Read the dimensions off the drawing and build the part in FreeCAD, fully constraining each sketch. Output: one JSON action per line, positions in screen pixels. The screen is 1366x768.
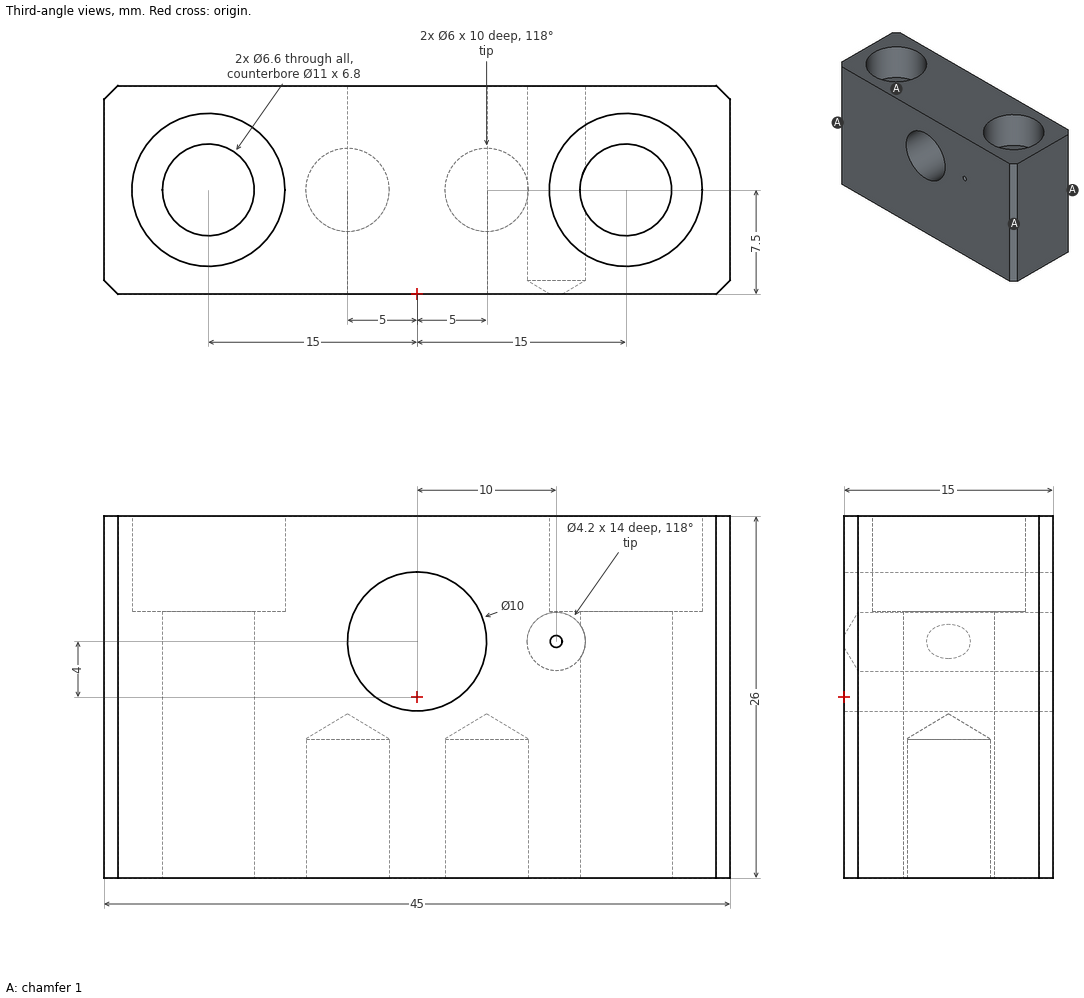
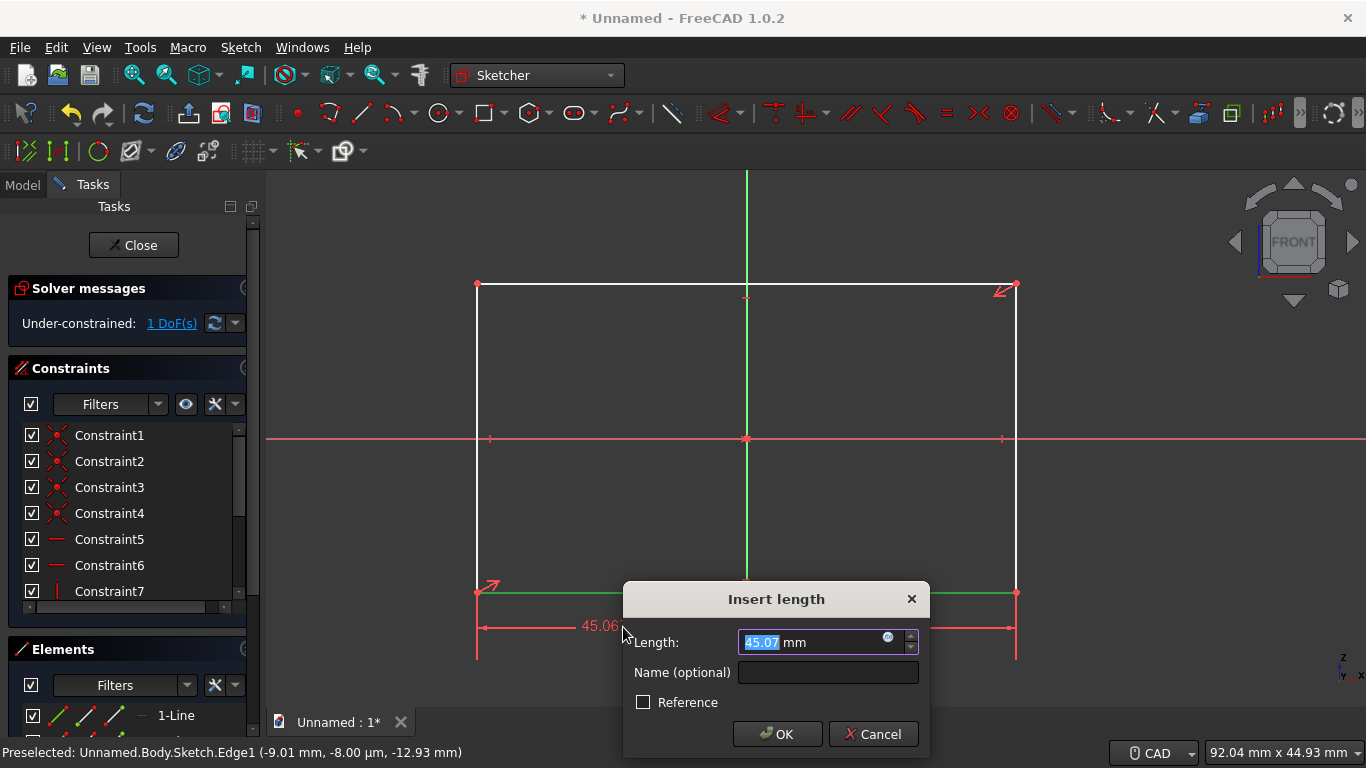
{"action": "type", "text": "45"}
{"action": "key", "text": "Return"}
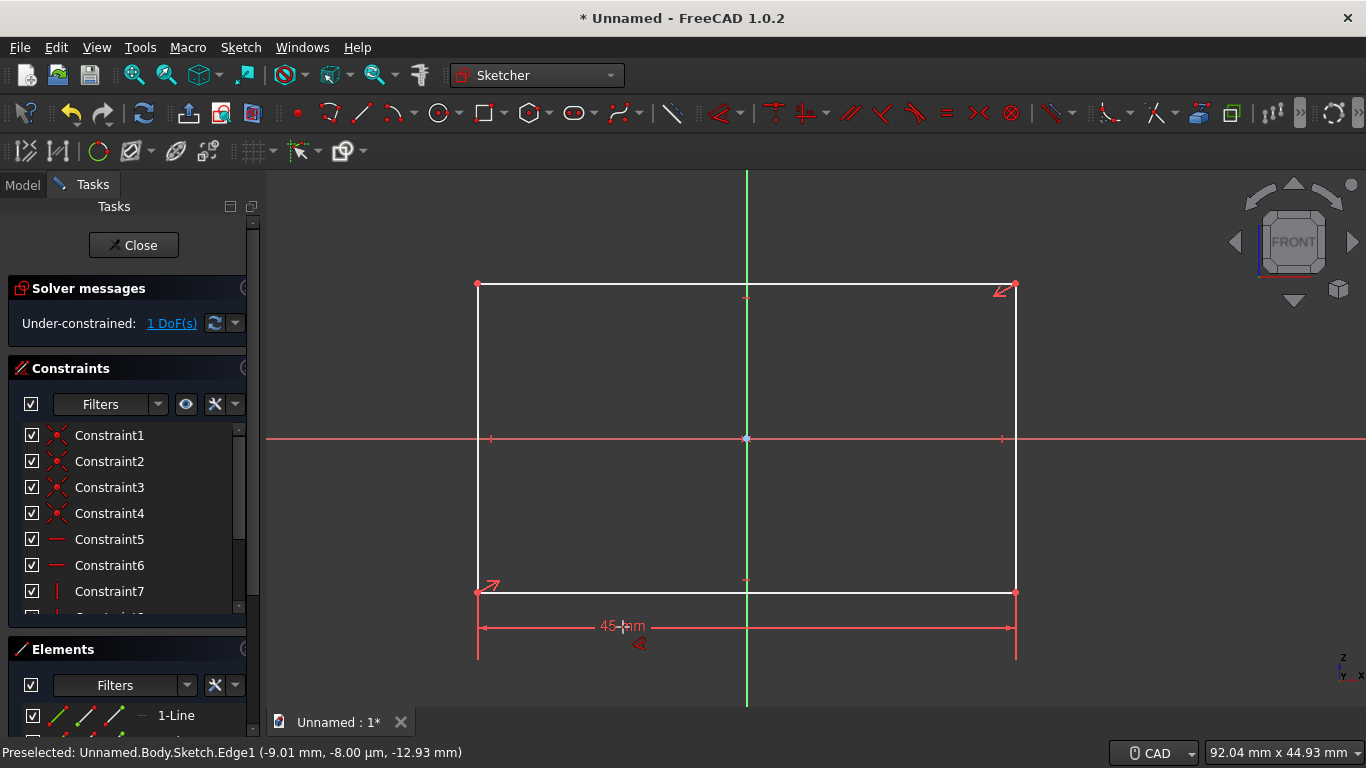
{"action": "left_click", "coordinate": [1016, 500]}
{"action": "left_click", "coordinate": [1050, 367]}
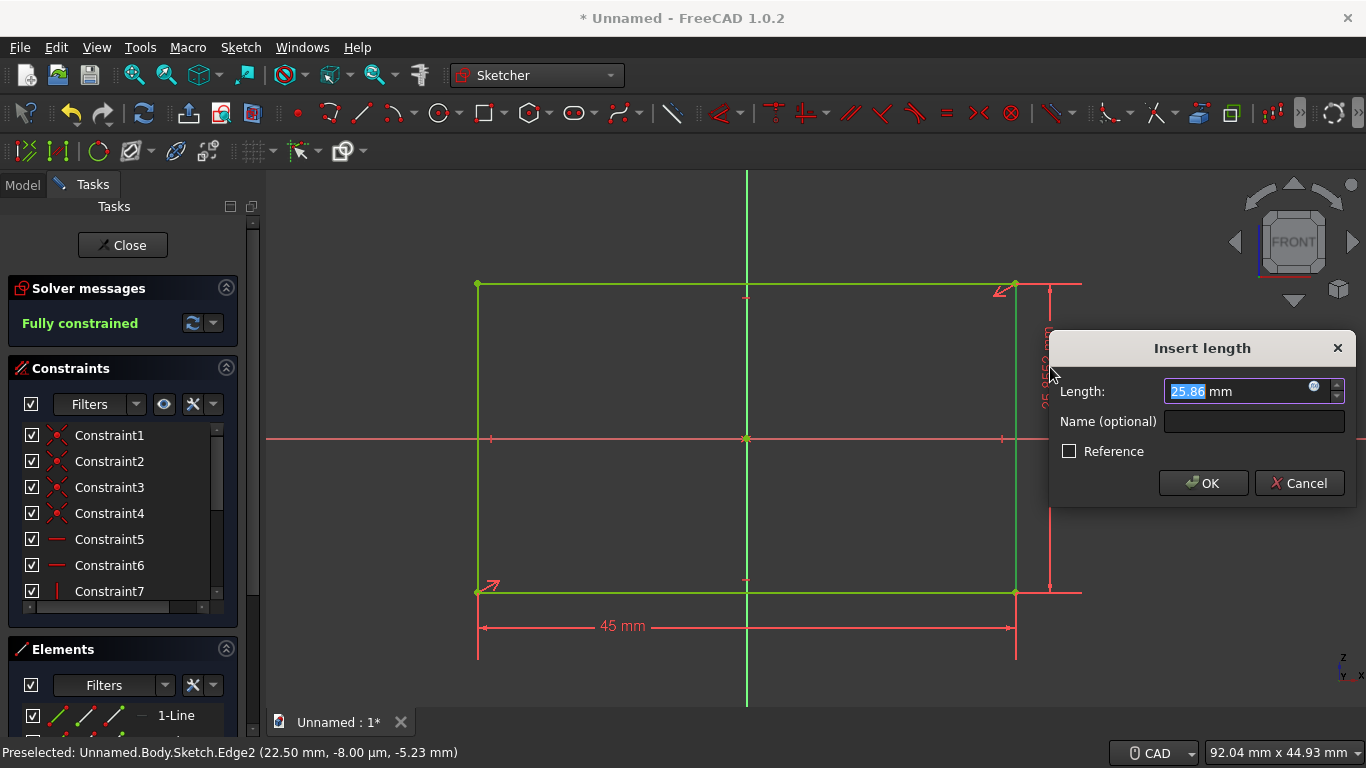
{"action": "type", "text": "26"}
{"action": "key", "text": "Return"}
{"action": "key", "text": "Escape"}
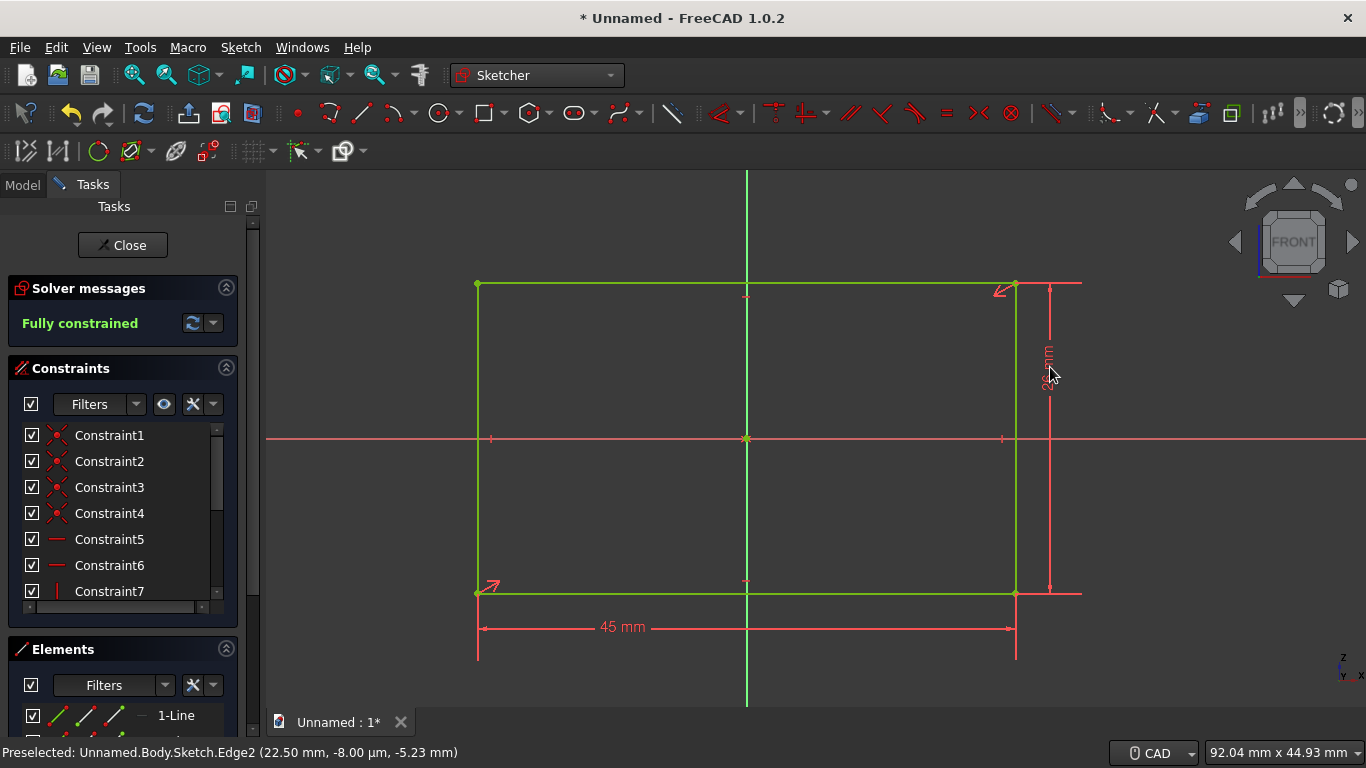
{"action": "left_click", "coordinate": [123, 245]}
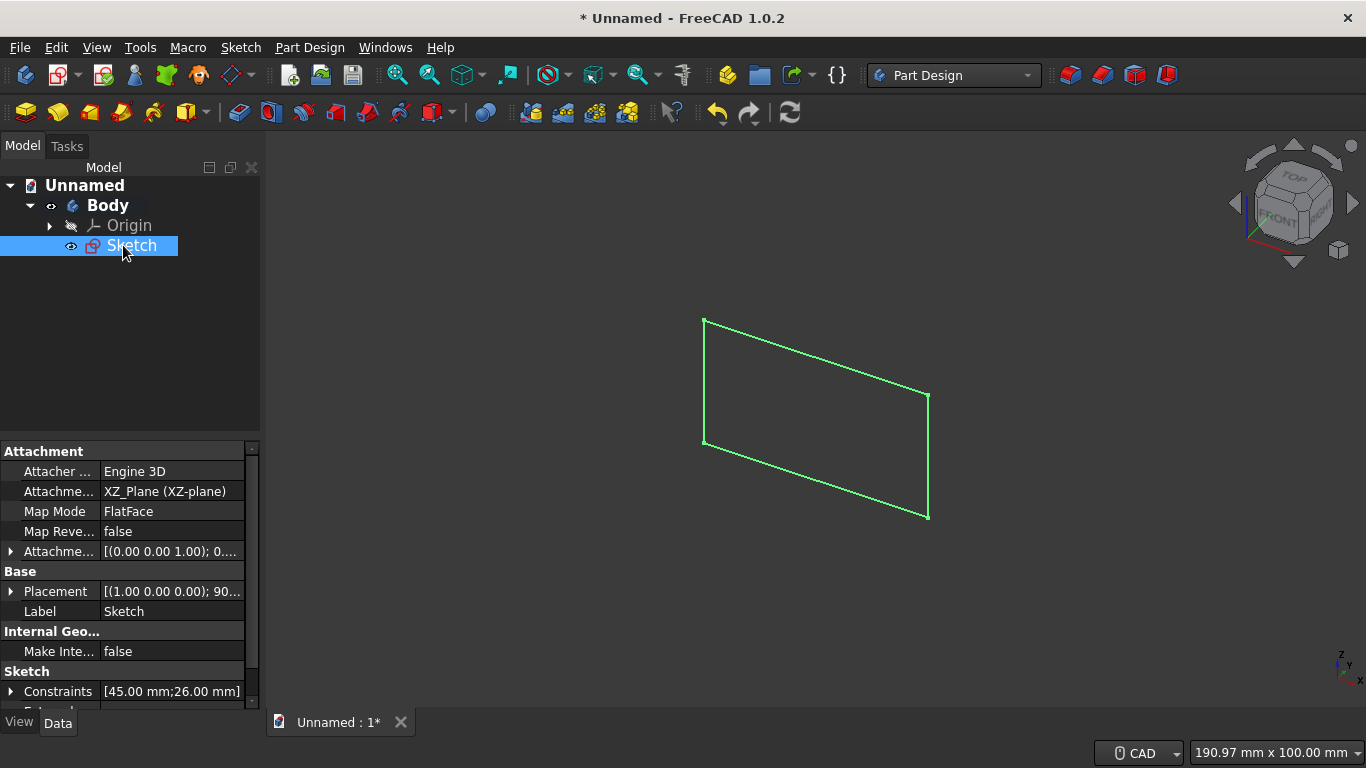
{"action": "left_click", "coordinate": [26, 112]}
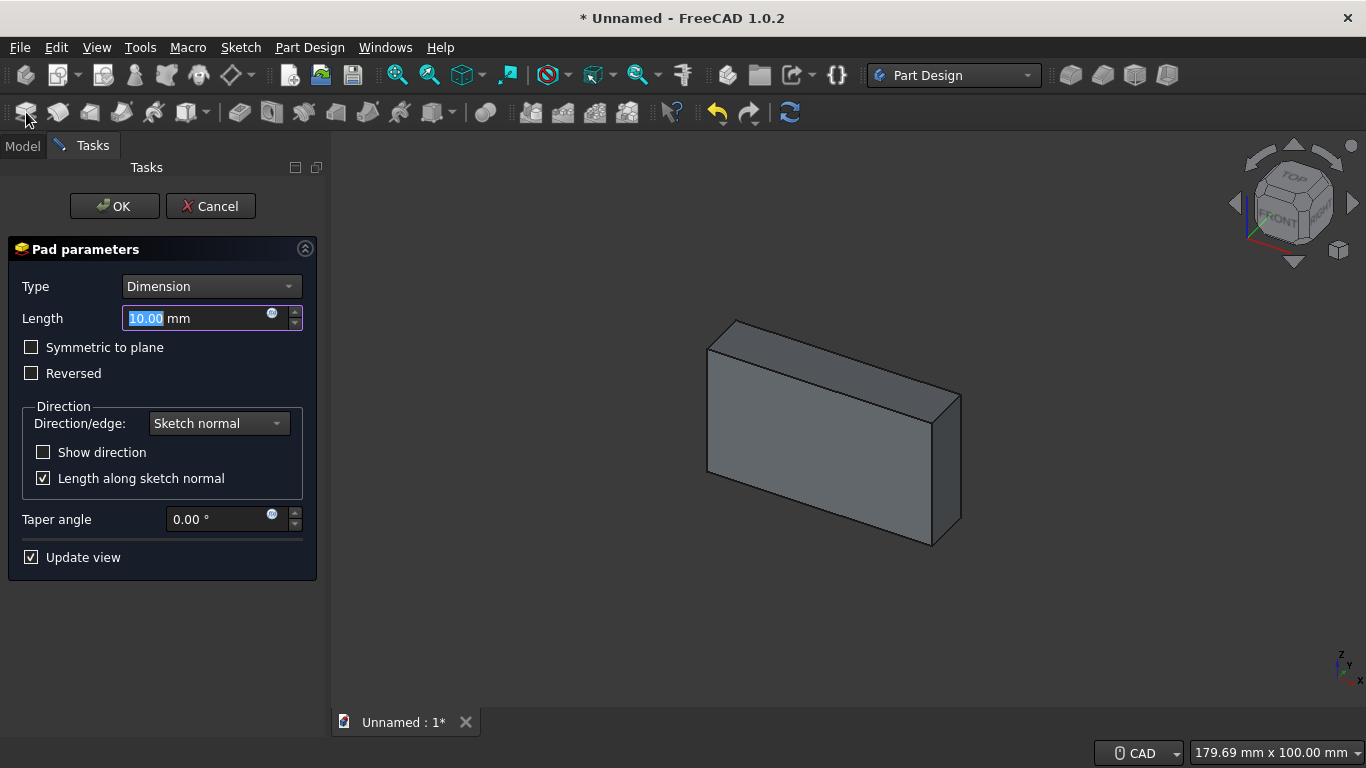
{"action": "type", "text": "15"}
{"action": "key", "text": "Tab"}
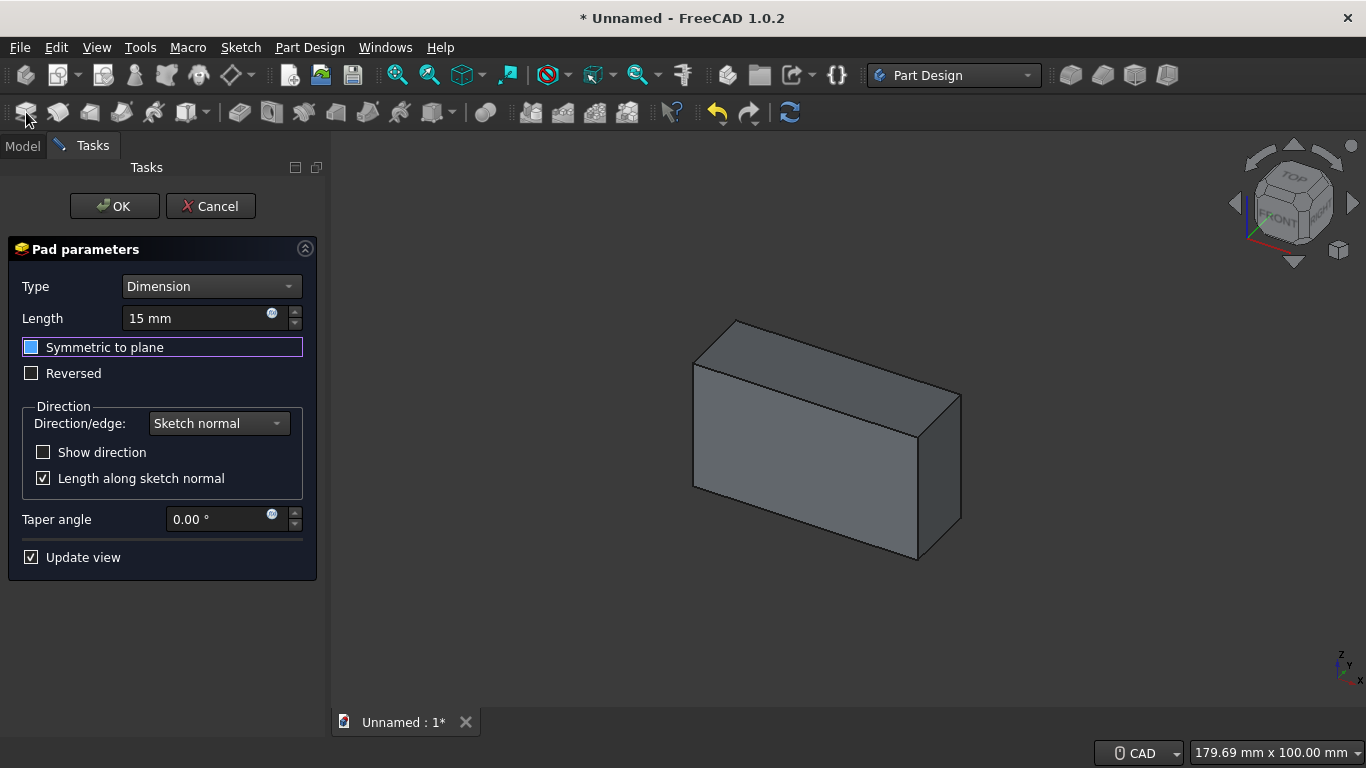
{"action": "left_click", "coordinate": [30, 373]}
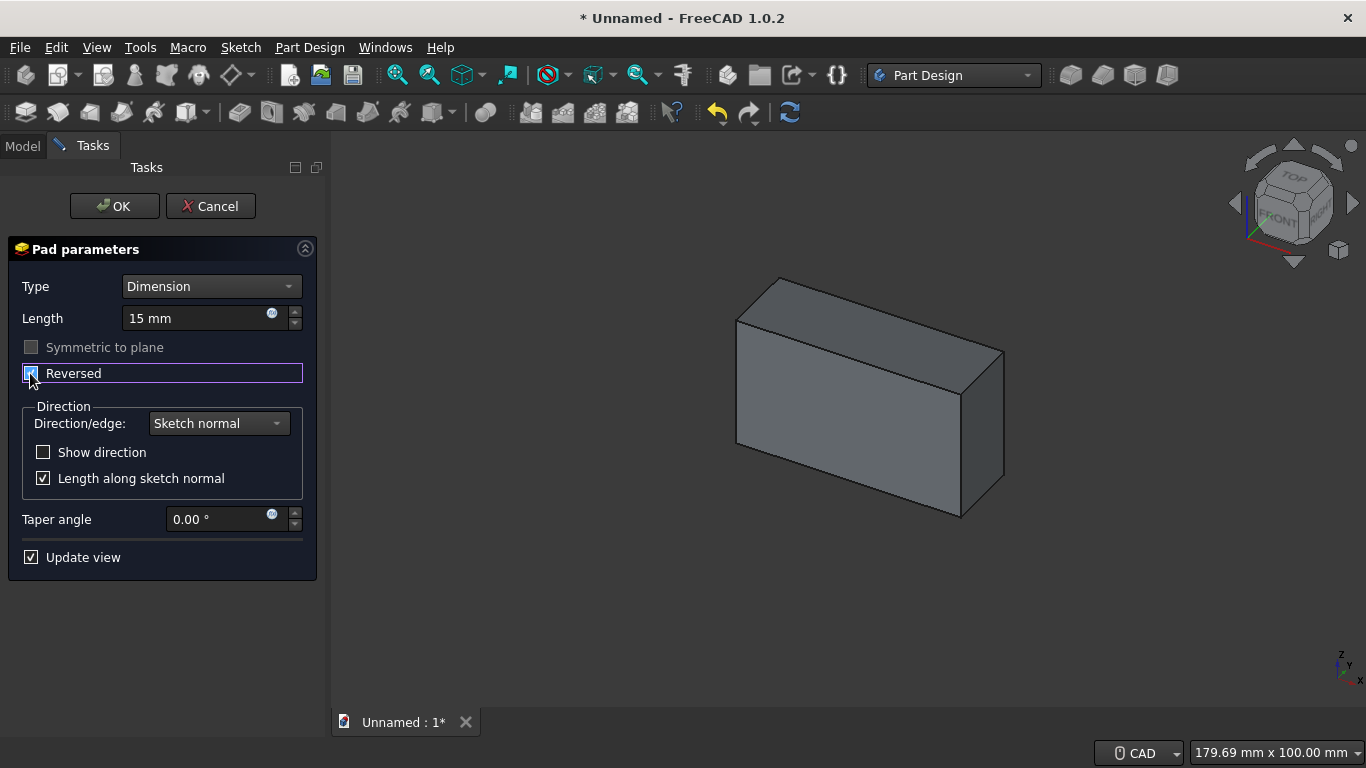
{"action": "left_click", "coordinate": [115, 206]}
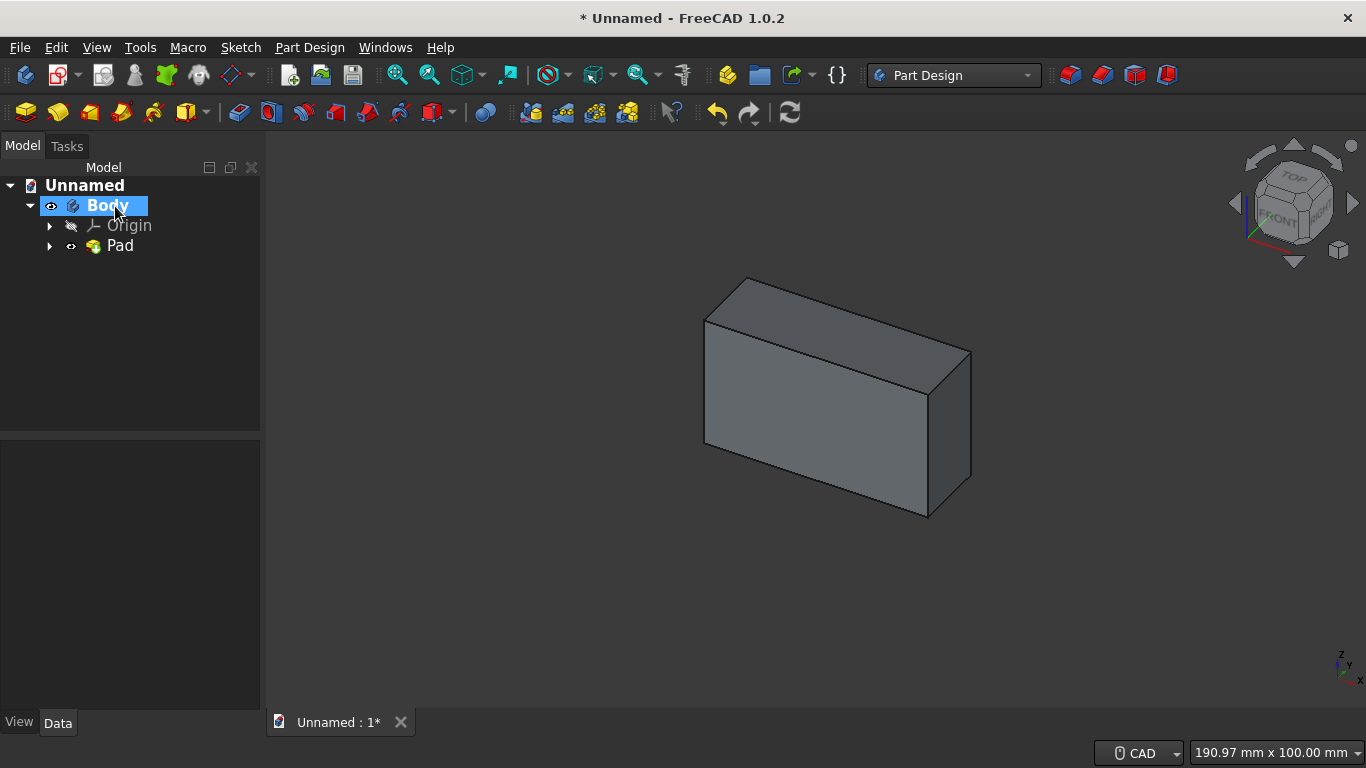
{"action": "left_click", "coordinate": [398, 76]}